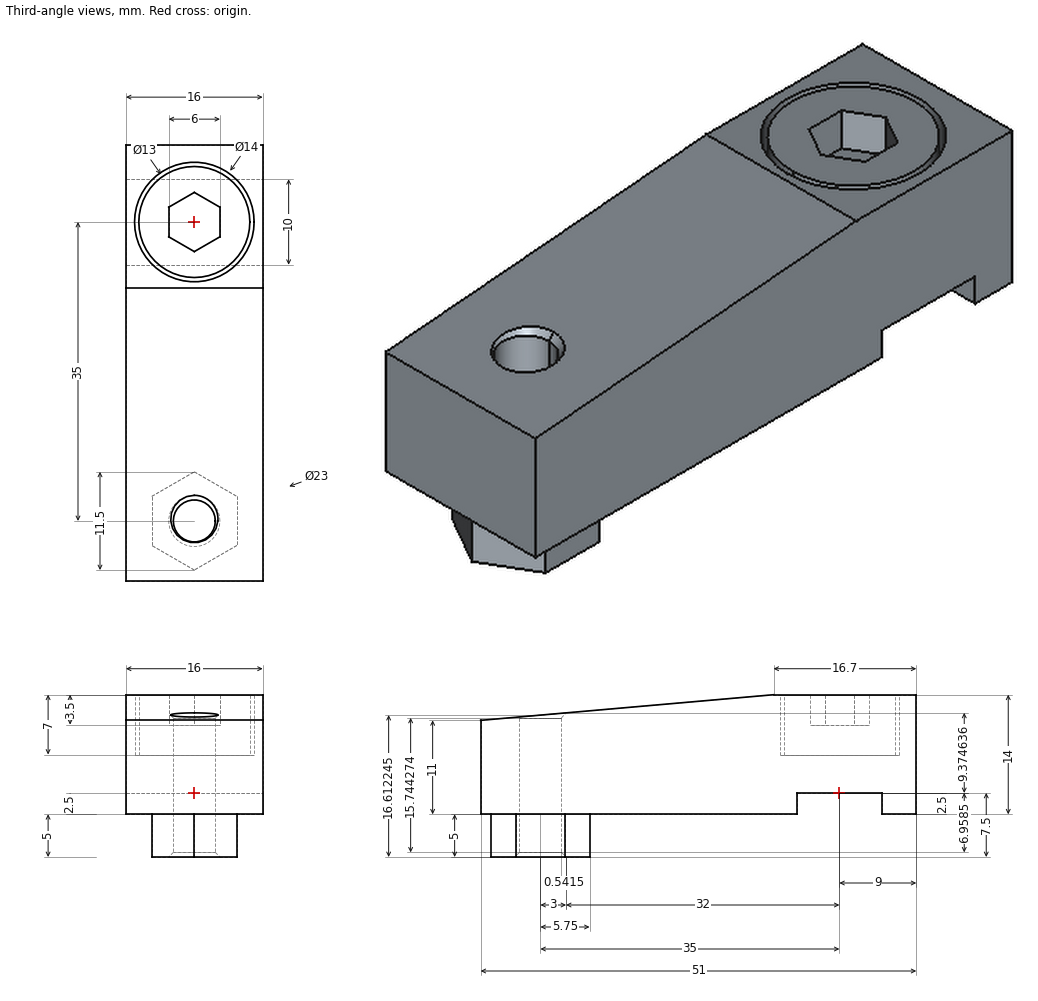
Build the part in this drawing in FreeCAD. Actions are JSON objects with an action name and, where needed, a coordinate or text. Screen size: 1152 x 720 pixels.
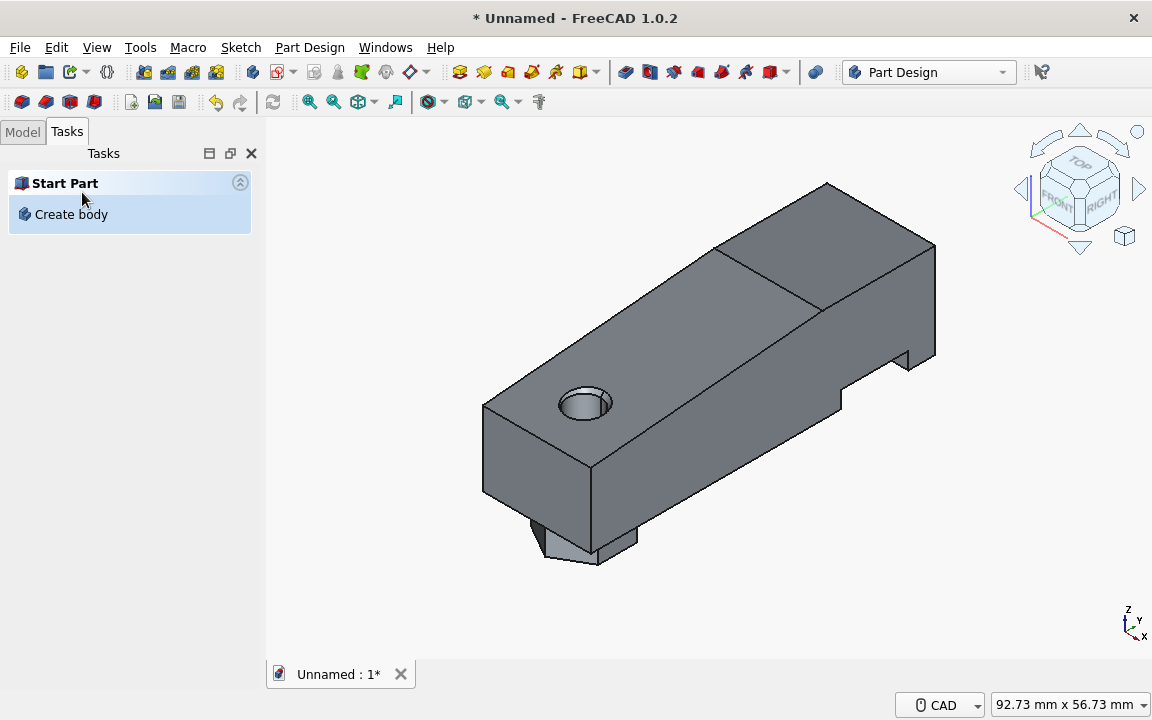
{"action": "left_click", "coordinate": [825, 246]}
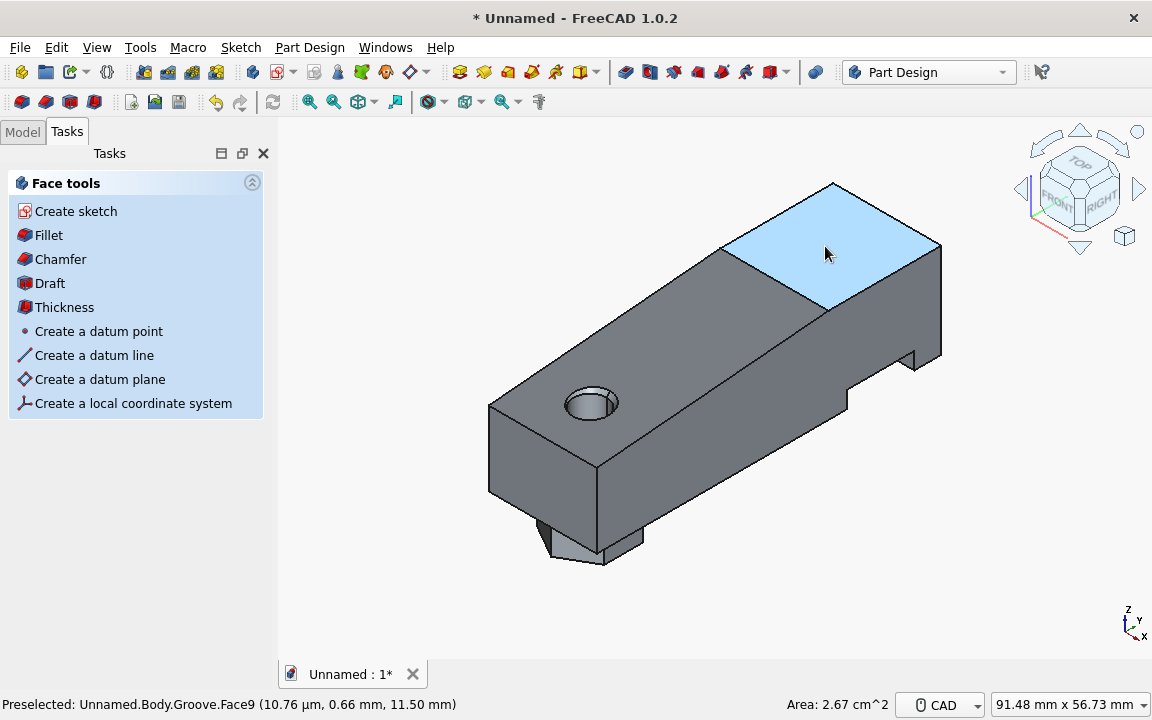
{"action": "left_click", "coordinate": [278, 72]}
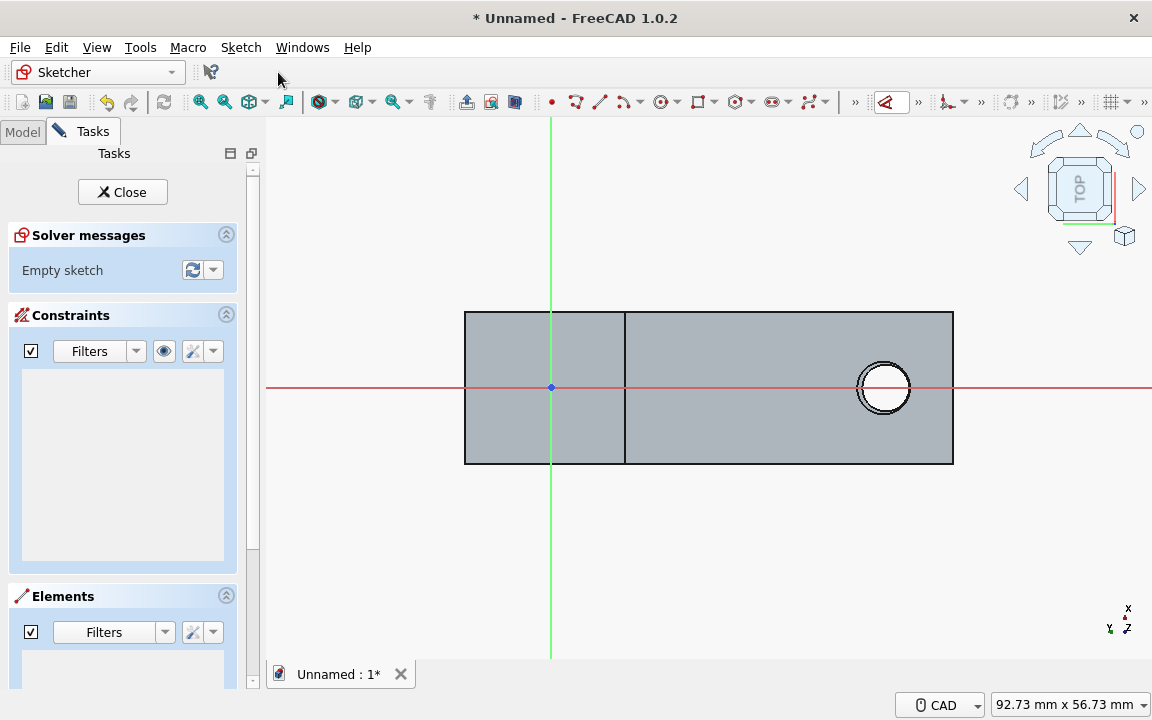
{"action": "scroll", "coordinate": [499, 388], "scroll_direction": "up", "scroll_amount": 5}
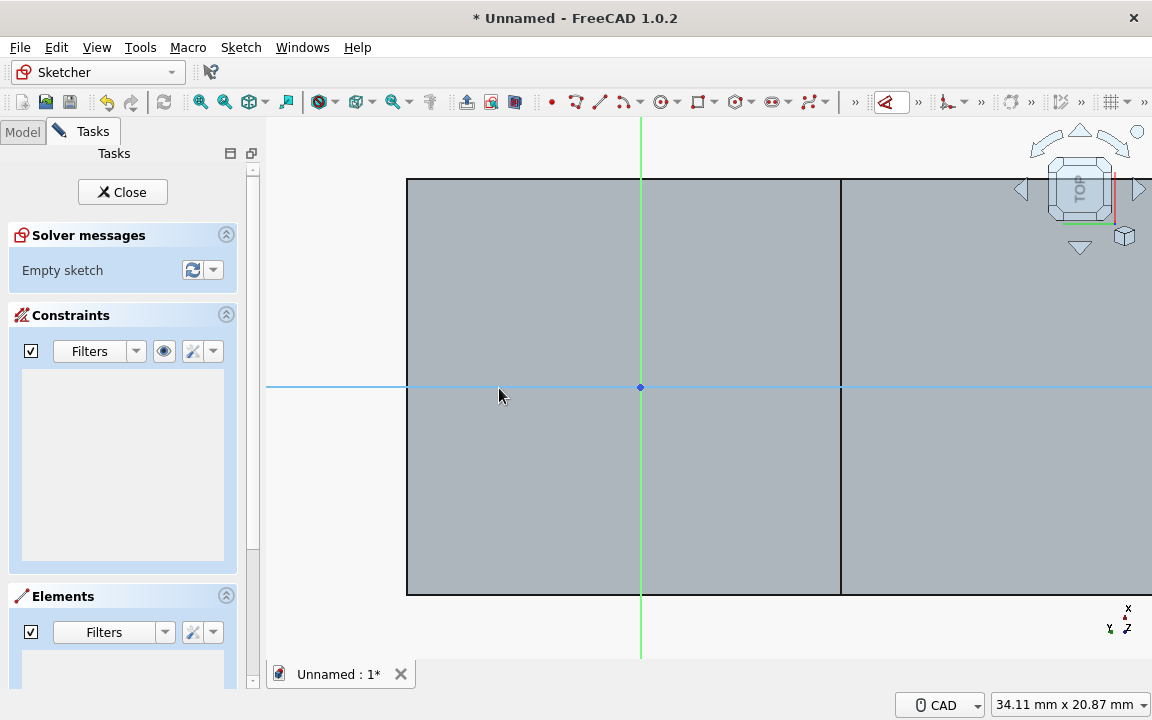
{"action": "left_click", "coordinate": [662, 102]}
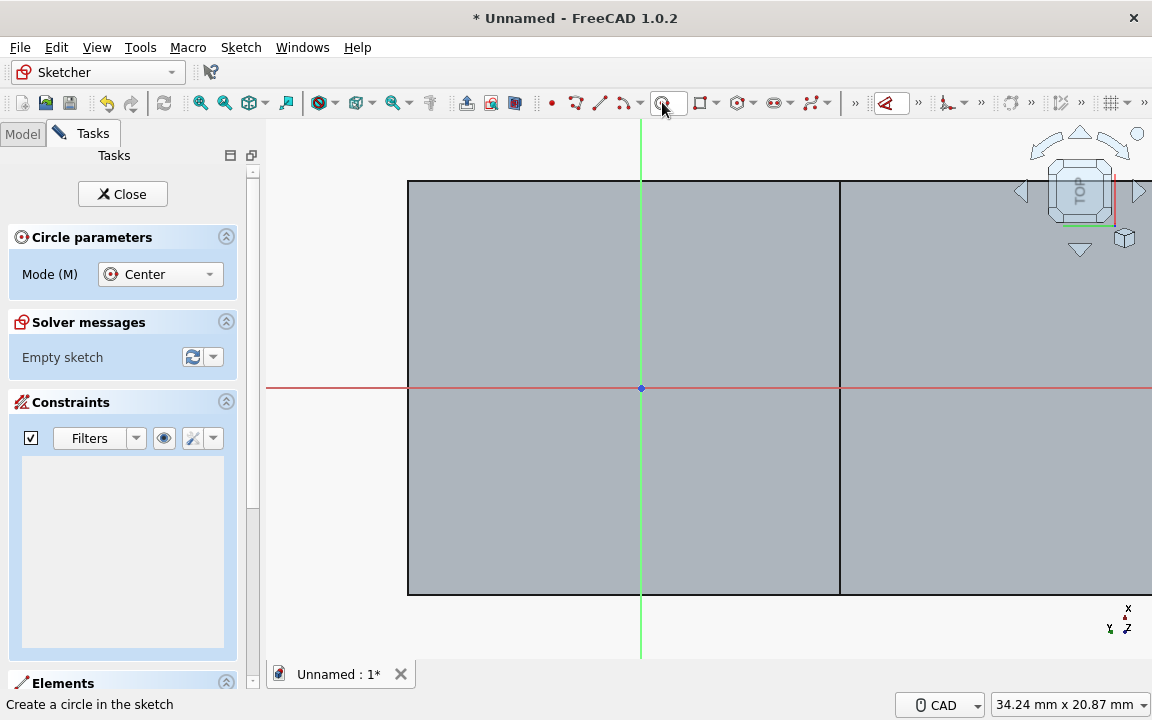
{"action": "left_click", "coordinate": [641, 388]}
{"action": "left_click", "coordinate": [769, 260]}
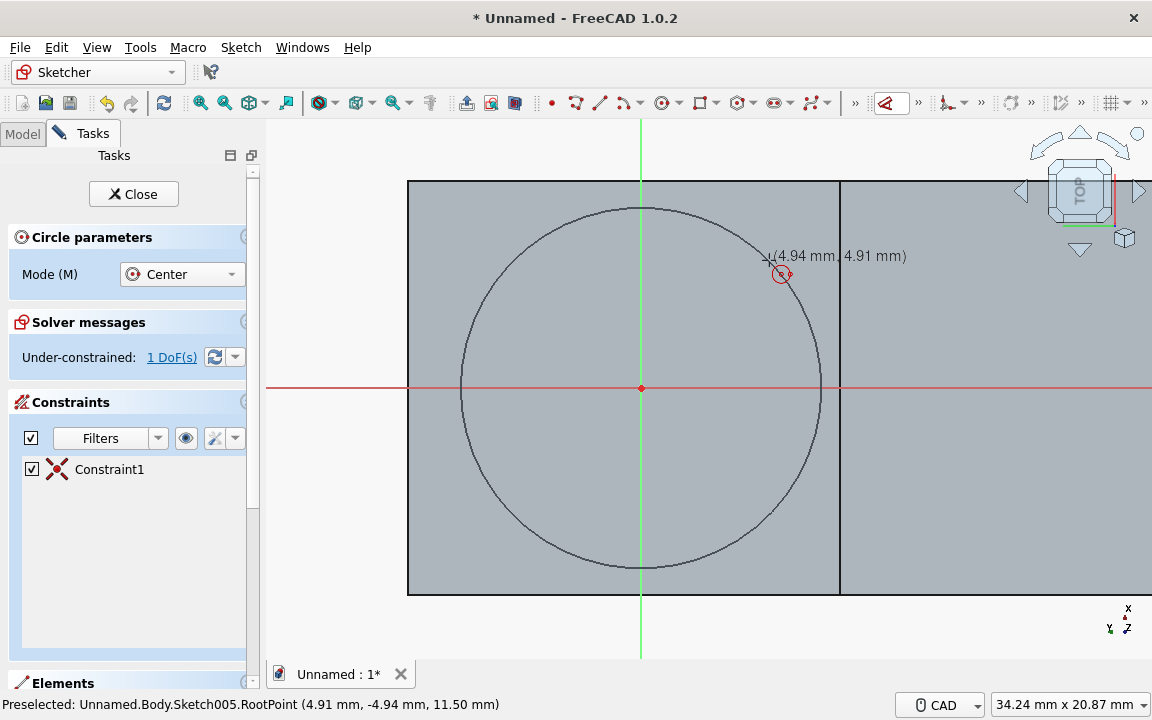
{"action": "left_click", "coordinate": [641, 388]}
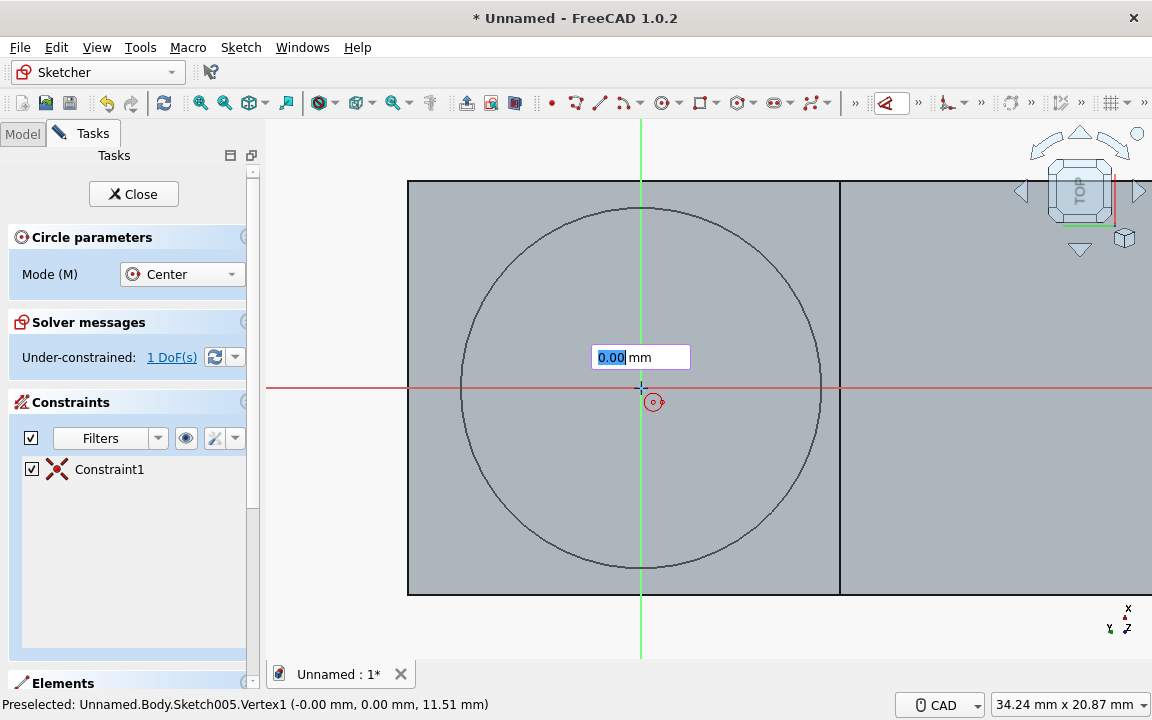
{"action": "scroll", "coordinate": [760, 269], "scroll_direction": "up", "scroll_amount": 2}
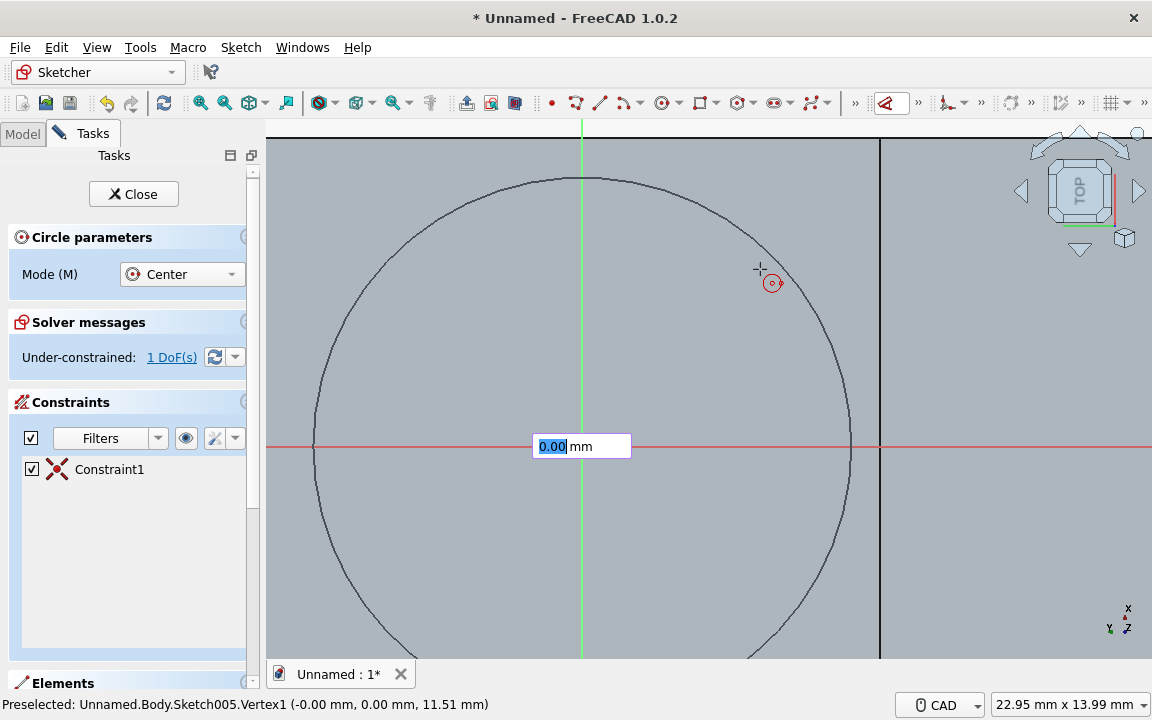
{"action": "left_click", "coordinate": [760, 269]}
{"action": "key", "text": "Escape"}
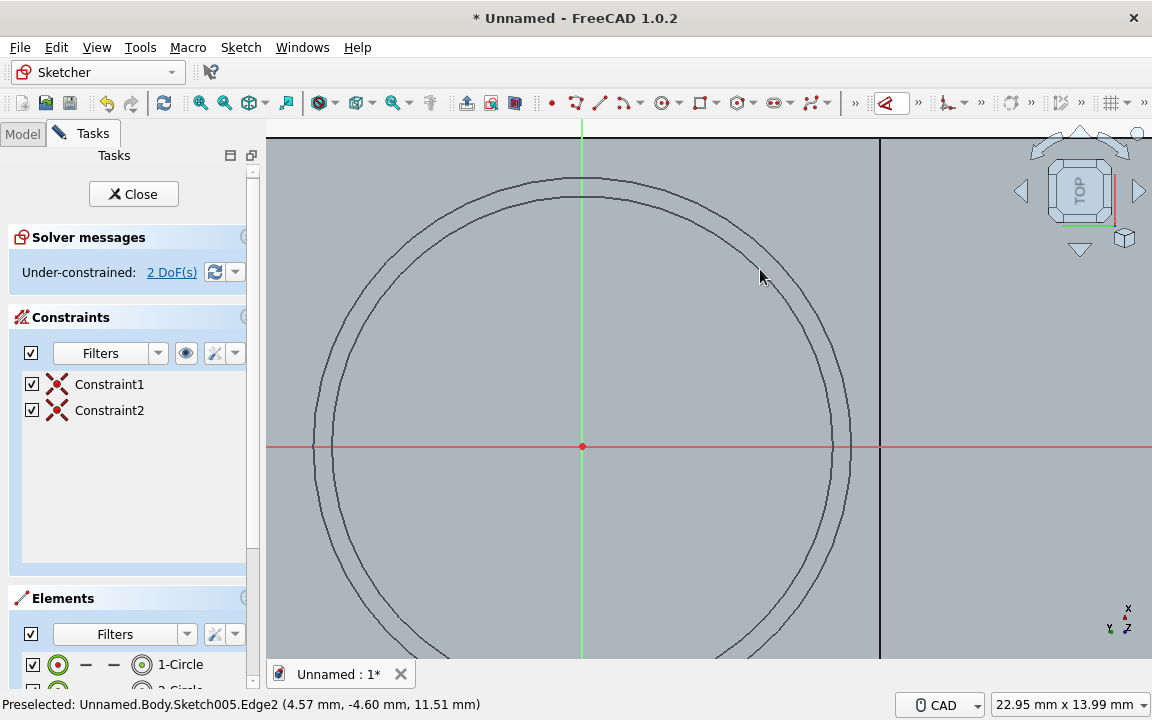
{"action": "left_click", "coordinate": [772, 256]}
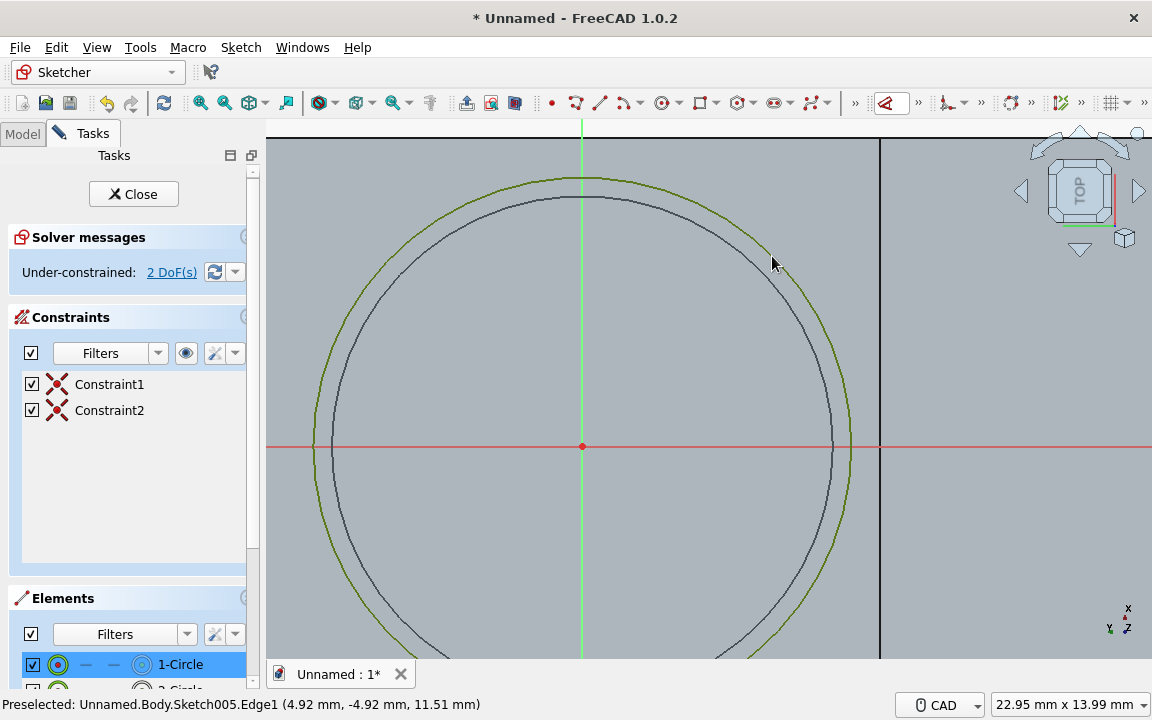
{"action": "key", "text": "k o"}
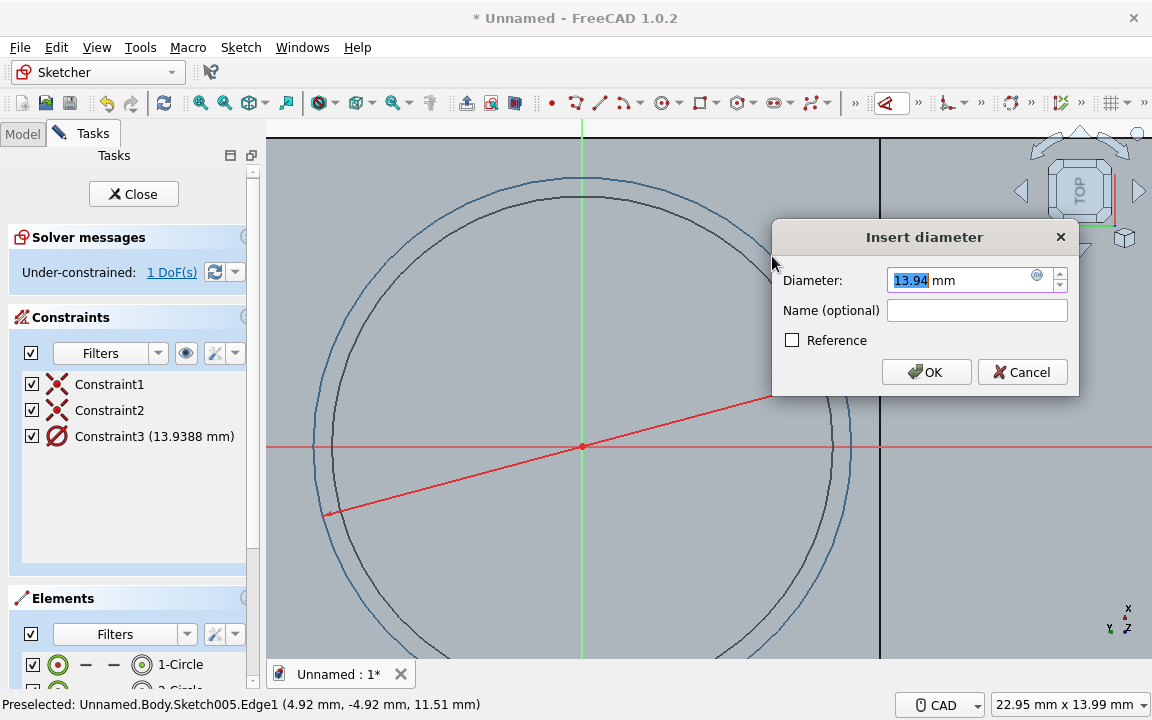
{"action": "type", "text": "14"}
{"action": "key", "text": "Return"}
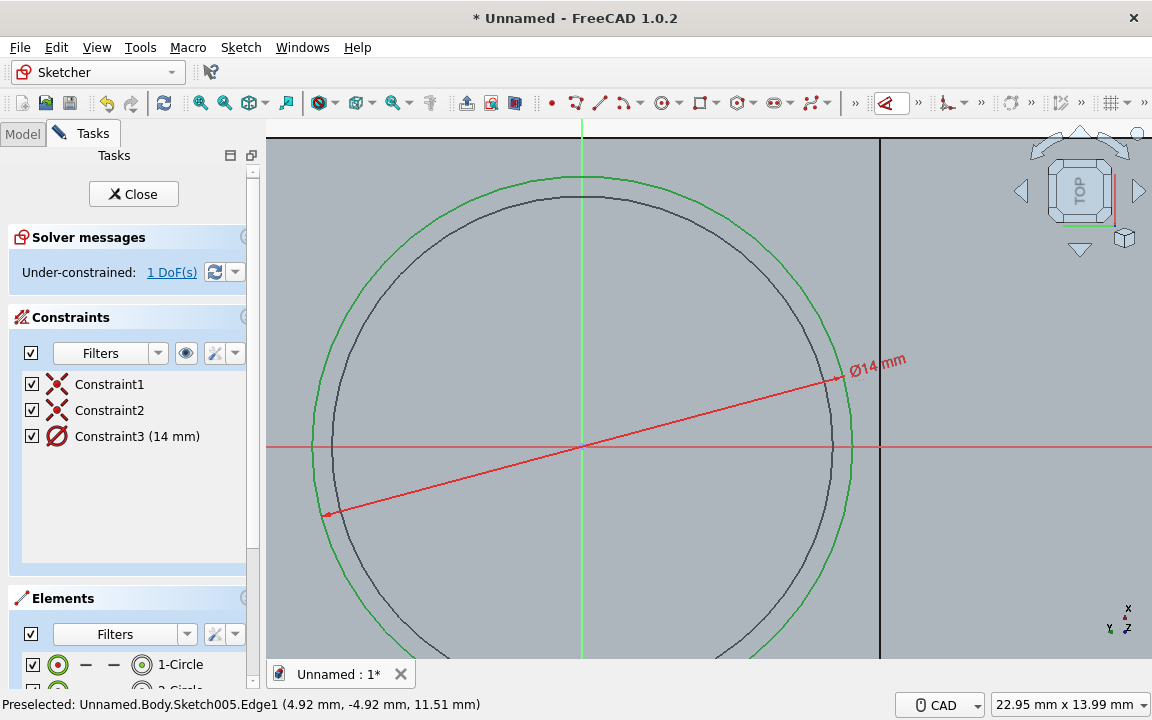
{"action": "left_click", "coordinate": [759, 269]}